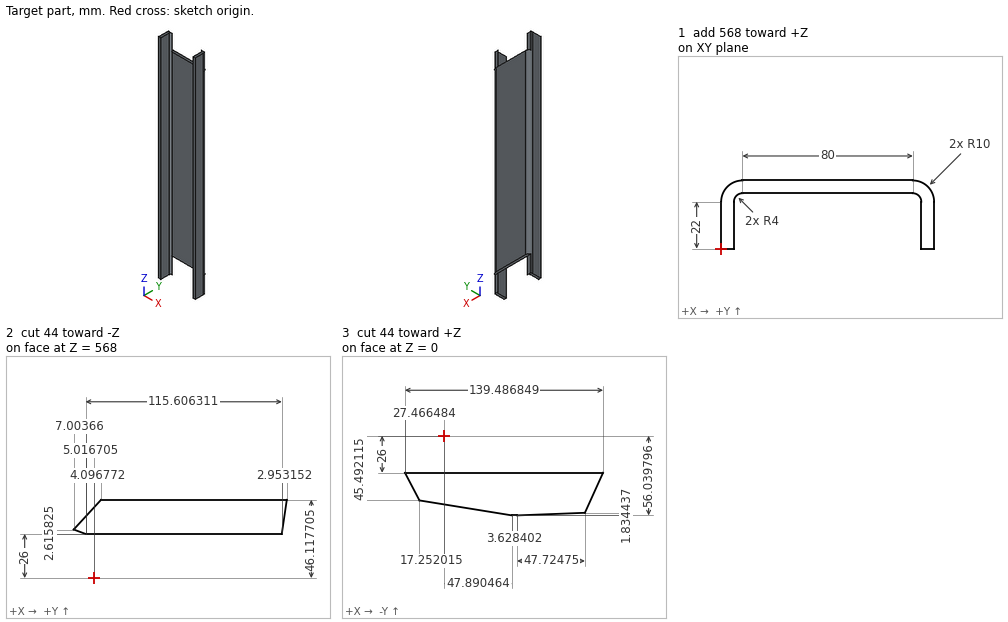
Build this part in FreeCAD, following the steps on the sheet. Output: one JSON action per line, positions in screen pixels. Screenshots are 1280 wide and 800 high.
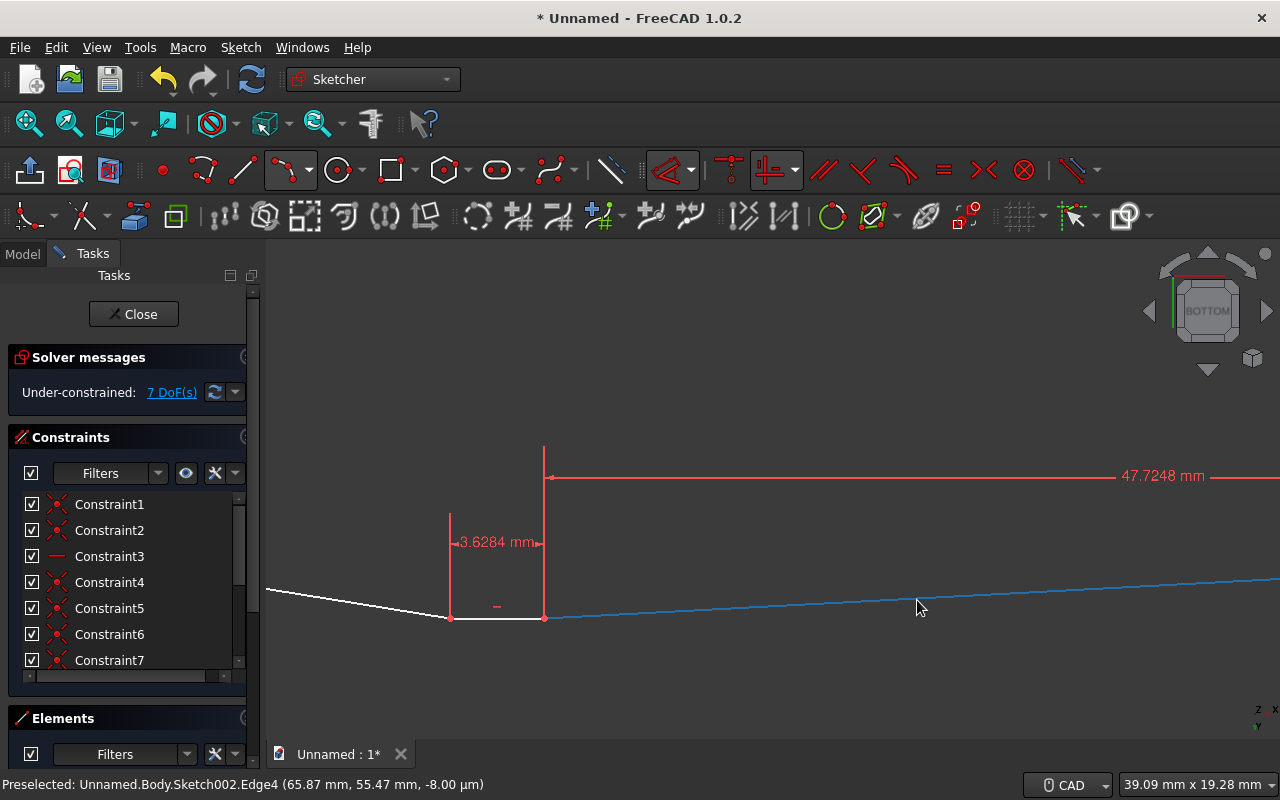
{"action": "left_click", "coordinate": [916, 599]}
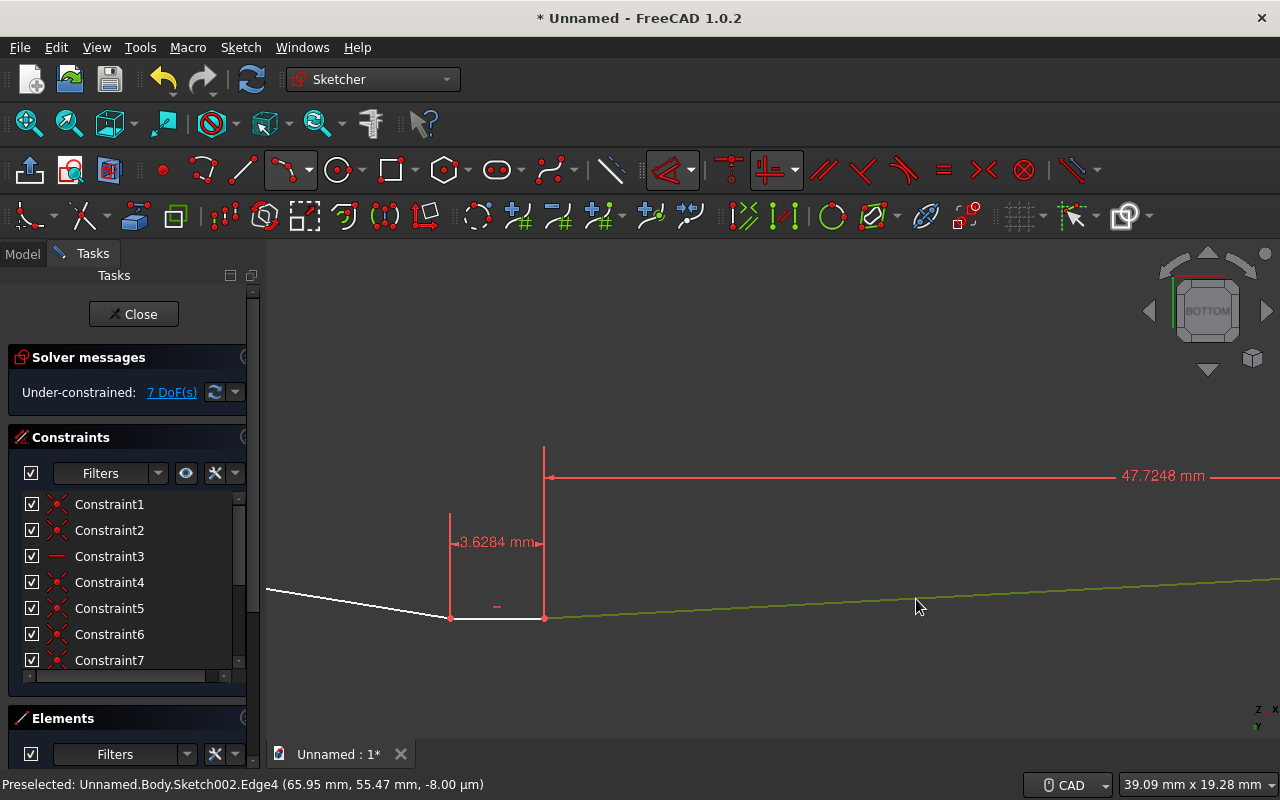
{"action": "left_click", "coordinate": [694, 170]}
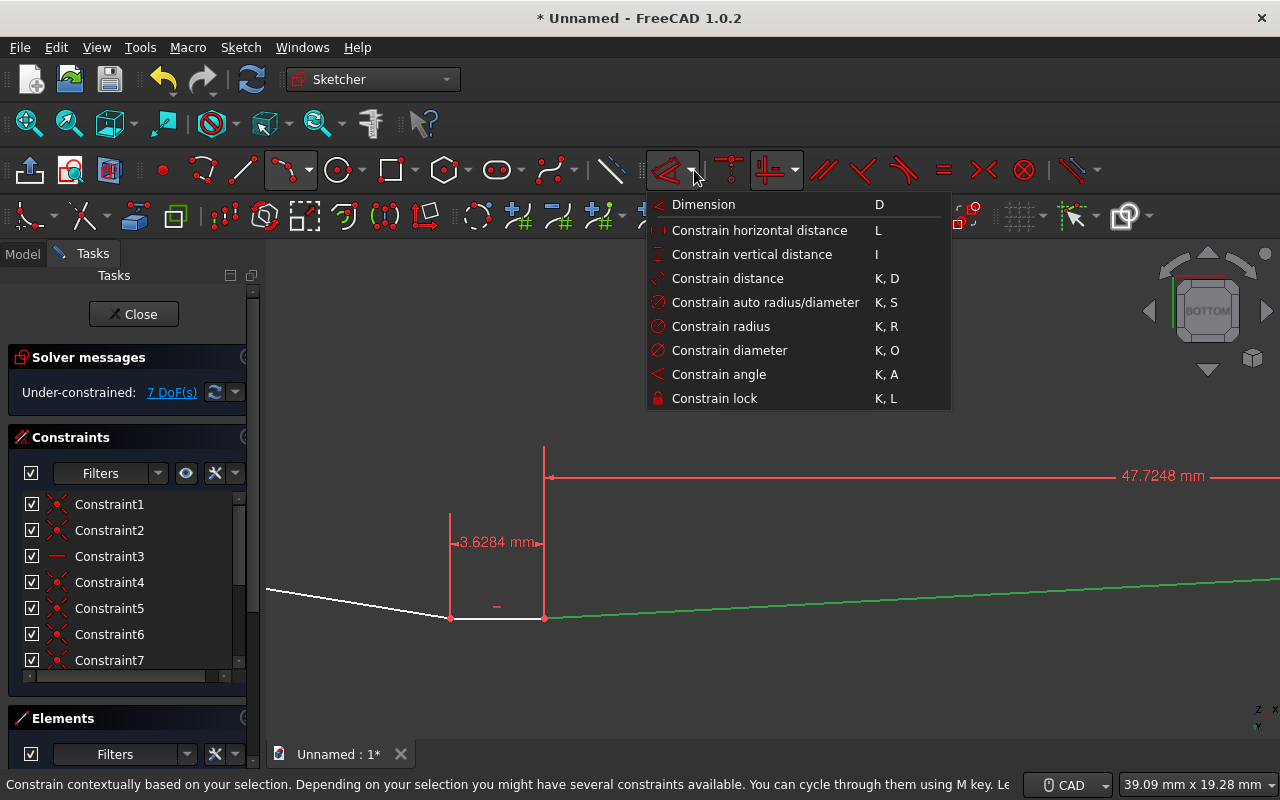
{"action": "left_click", "coordinate": [799, 254]}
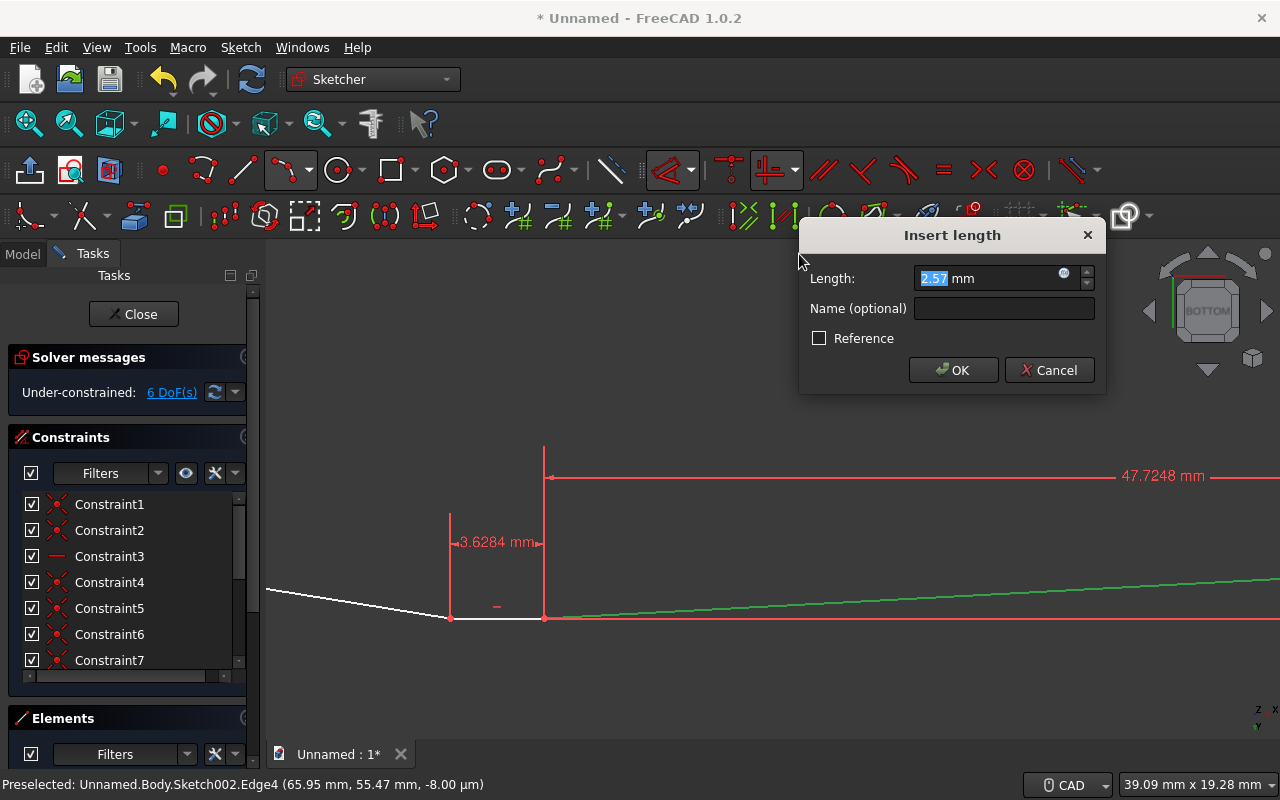
{"action": "type", "text": "1.834437"}
{"action": "key", "text": "Return"}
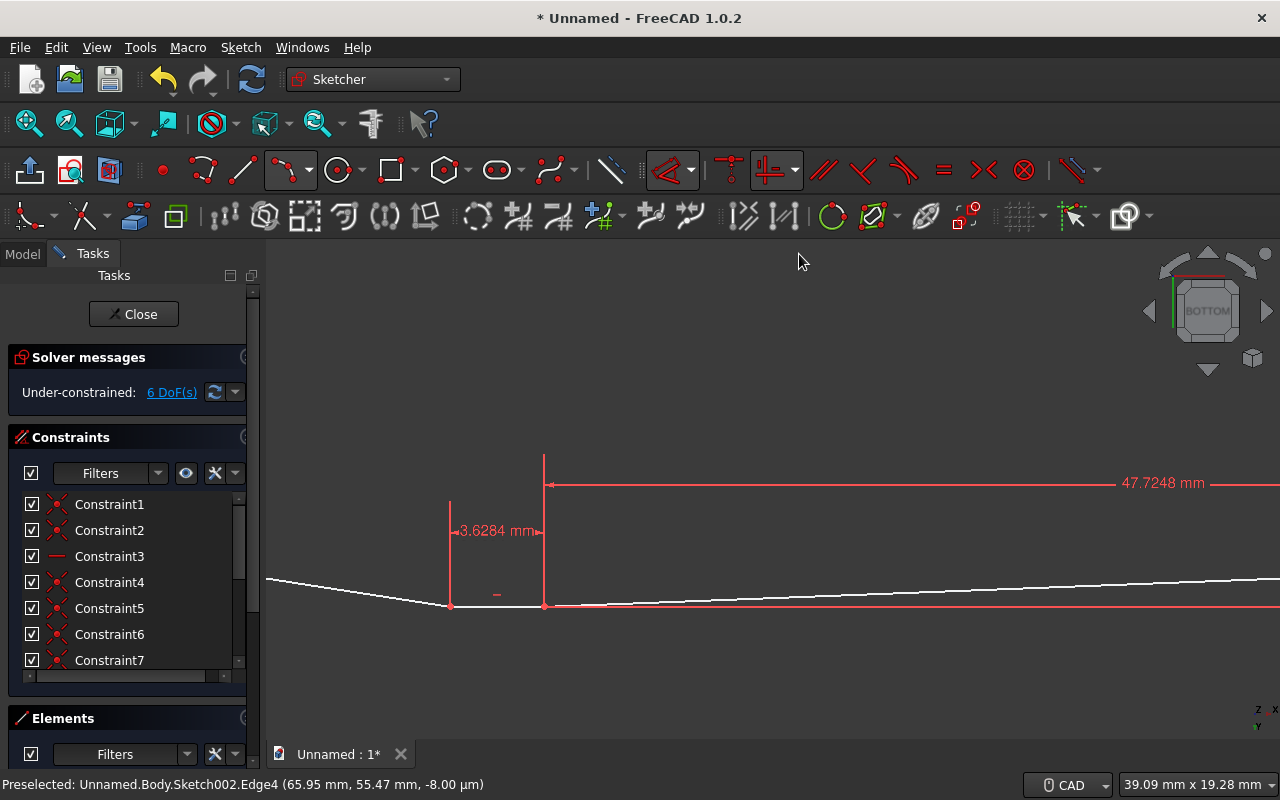
{"action": "scroll", "coordinate": [784, 608], "scroll_direction": "down", "scroll_amount": 9}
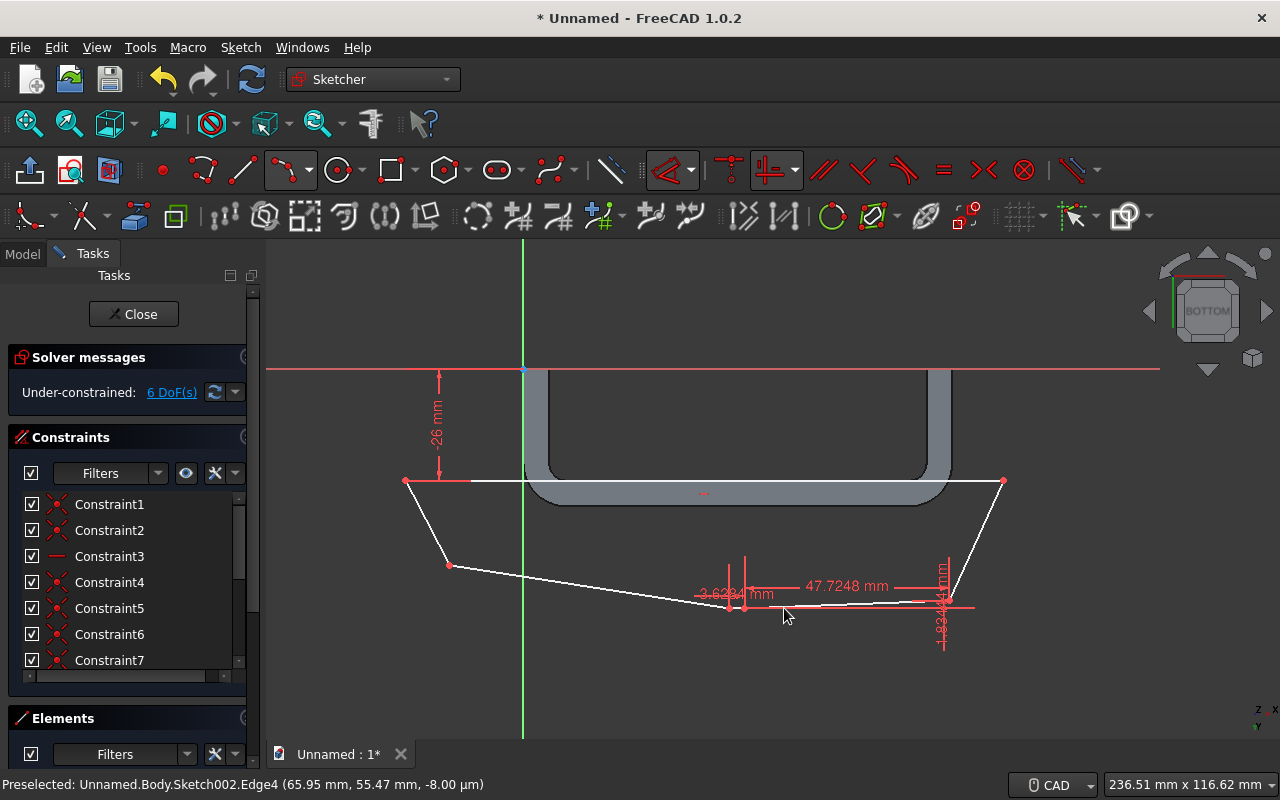
{"action": "left_click", "coordinate": [824, 481]}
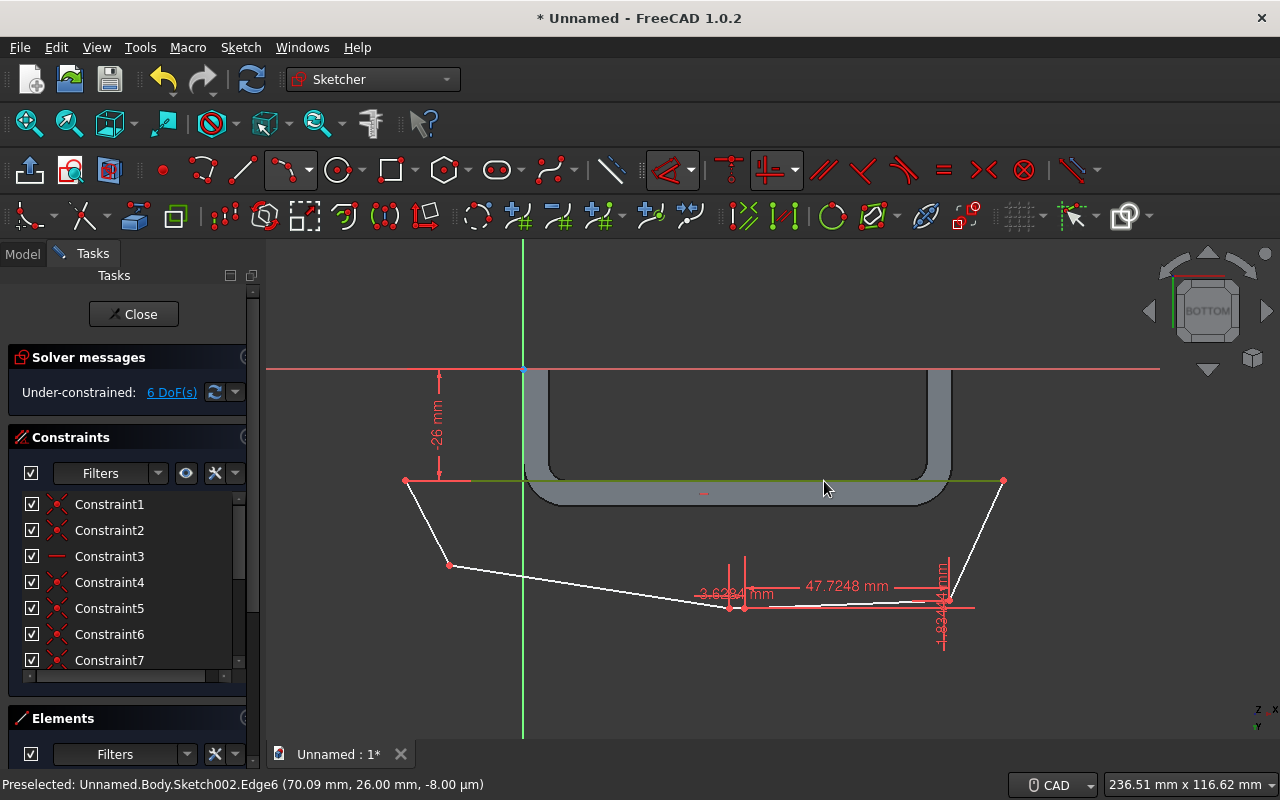
{"action": "key", "text": "l"}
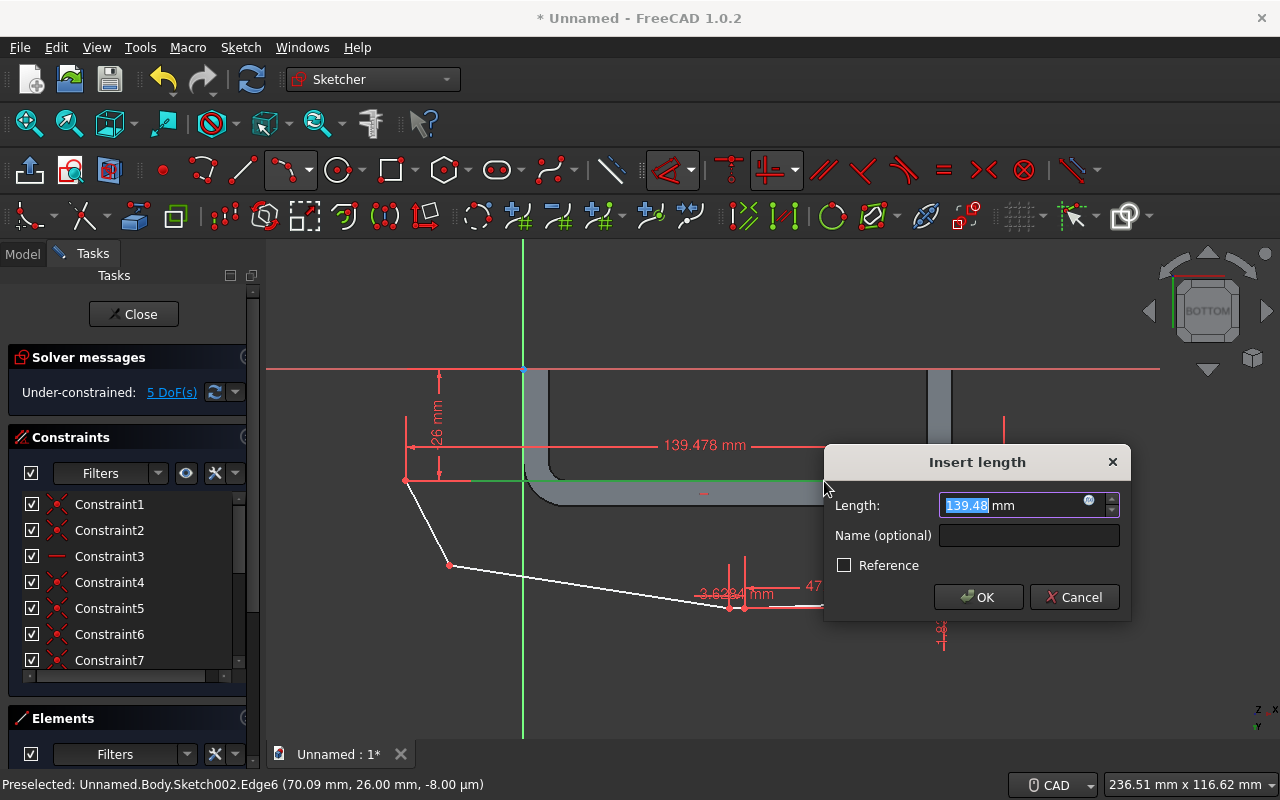
{"action": "type", "text": "139.486849"}
{"action": "key", "text": "Return"}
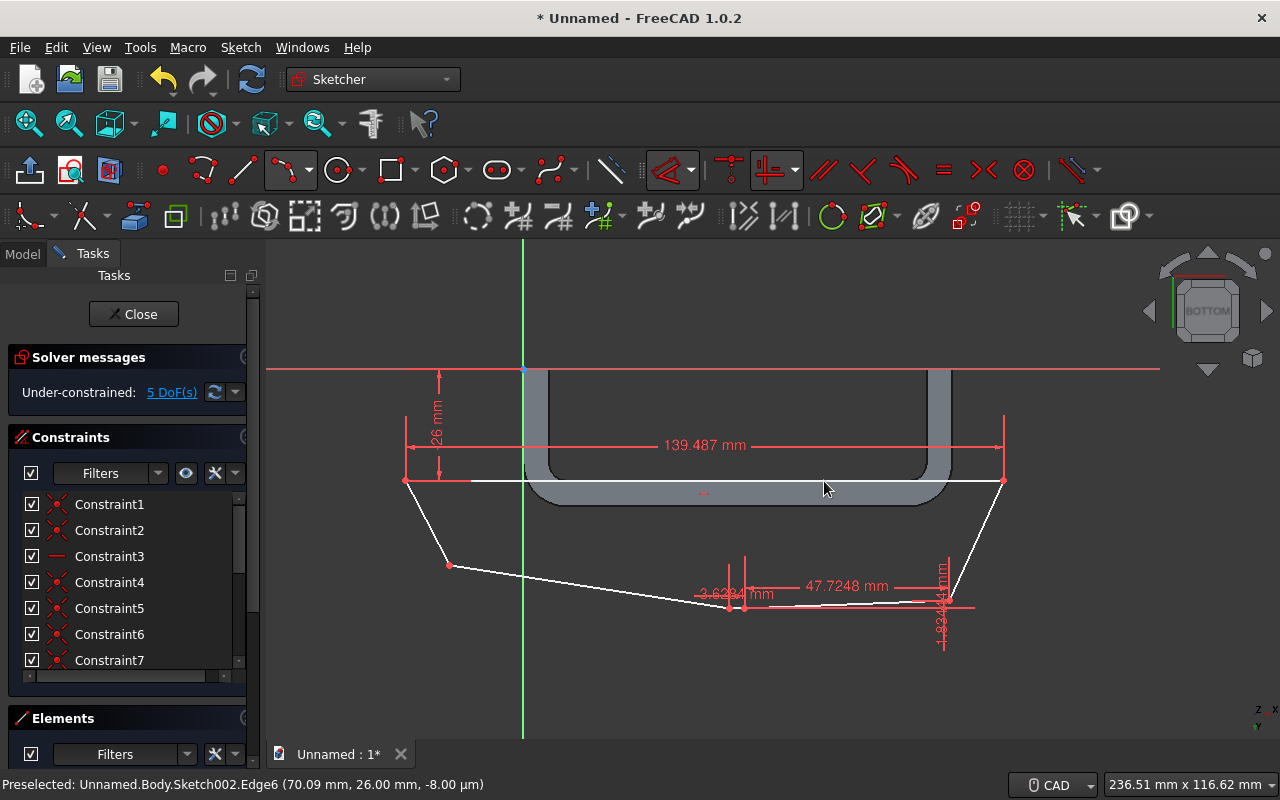
{"action": "left_click", "coordinate": [406, 481]}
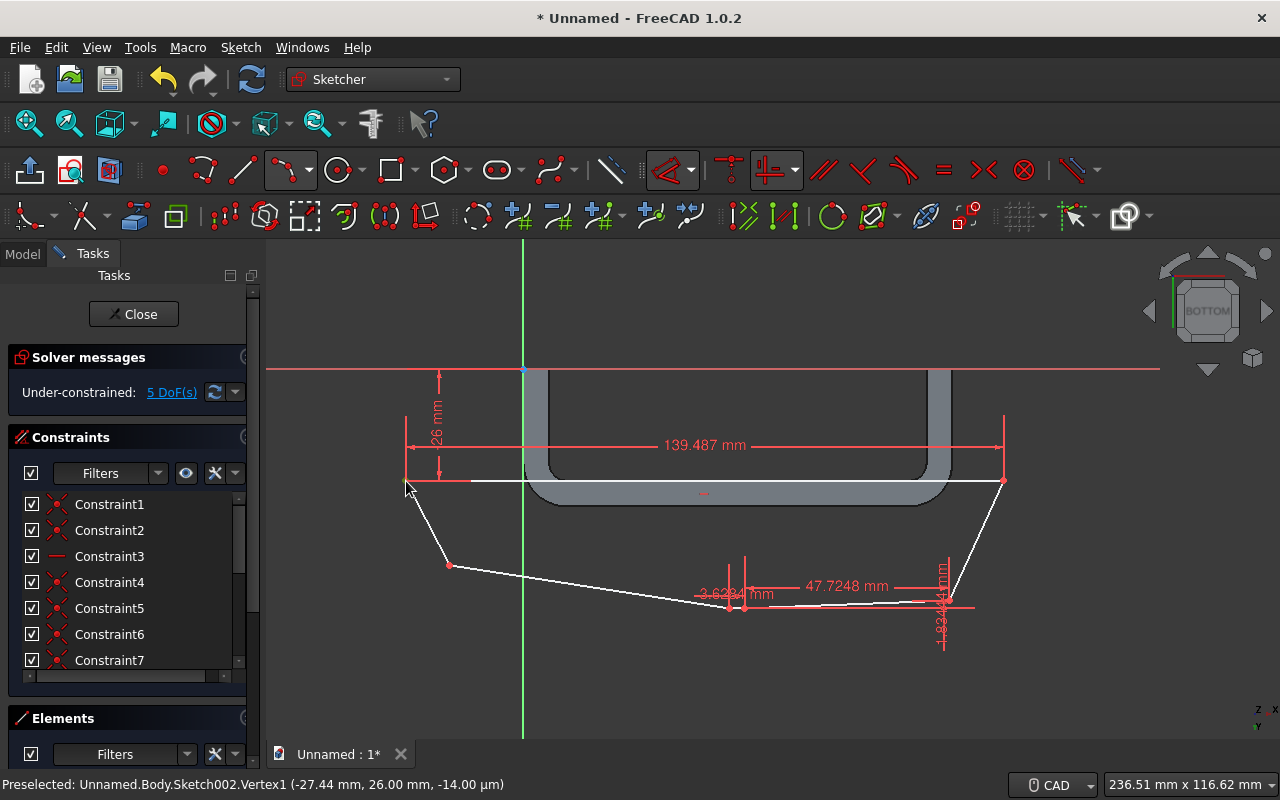
{"action": "left_click", "coordinate": [694, 170]}